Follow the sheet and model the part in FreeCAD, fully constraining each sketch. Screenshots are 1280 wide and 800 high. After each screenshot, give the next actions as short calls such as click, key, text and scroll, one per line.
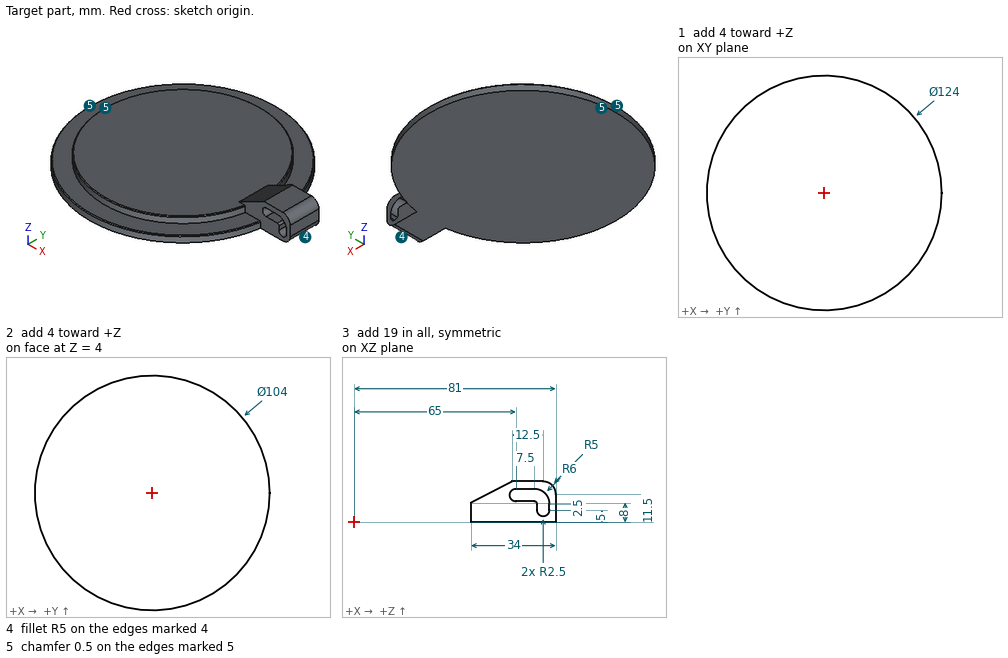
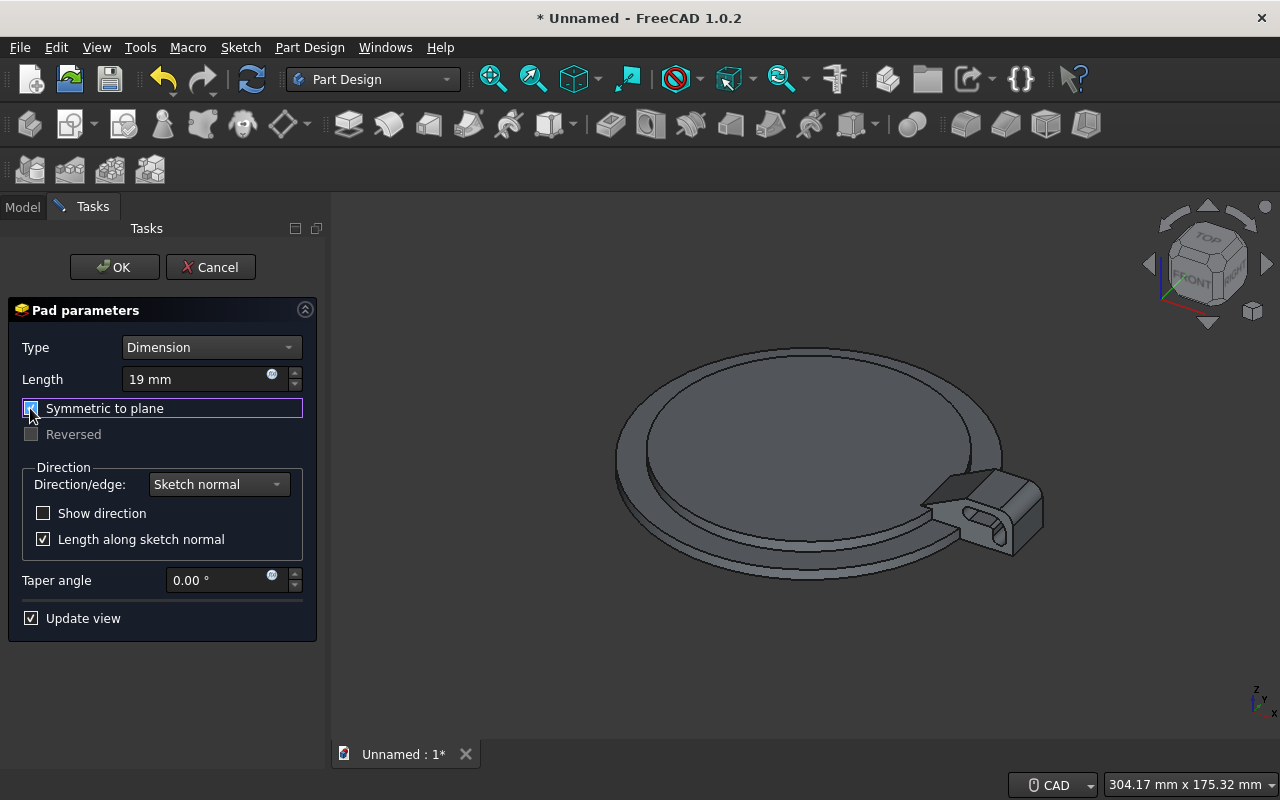
click(115, 267)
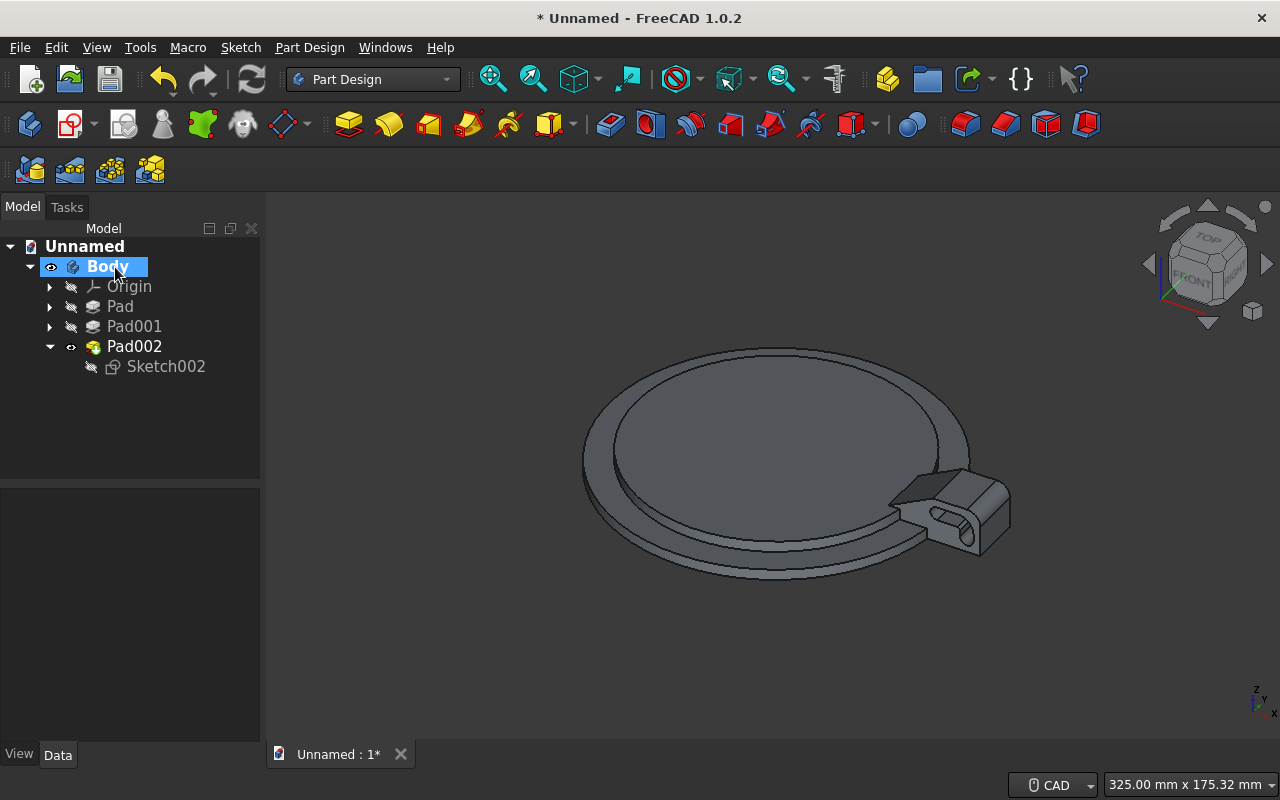
key(0)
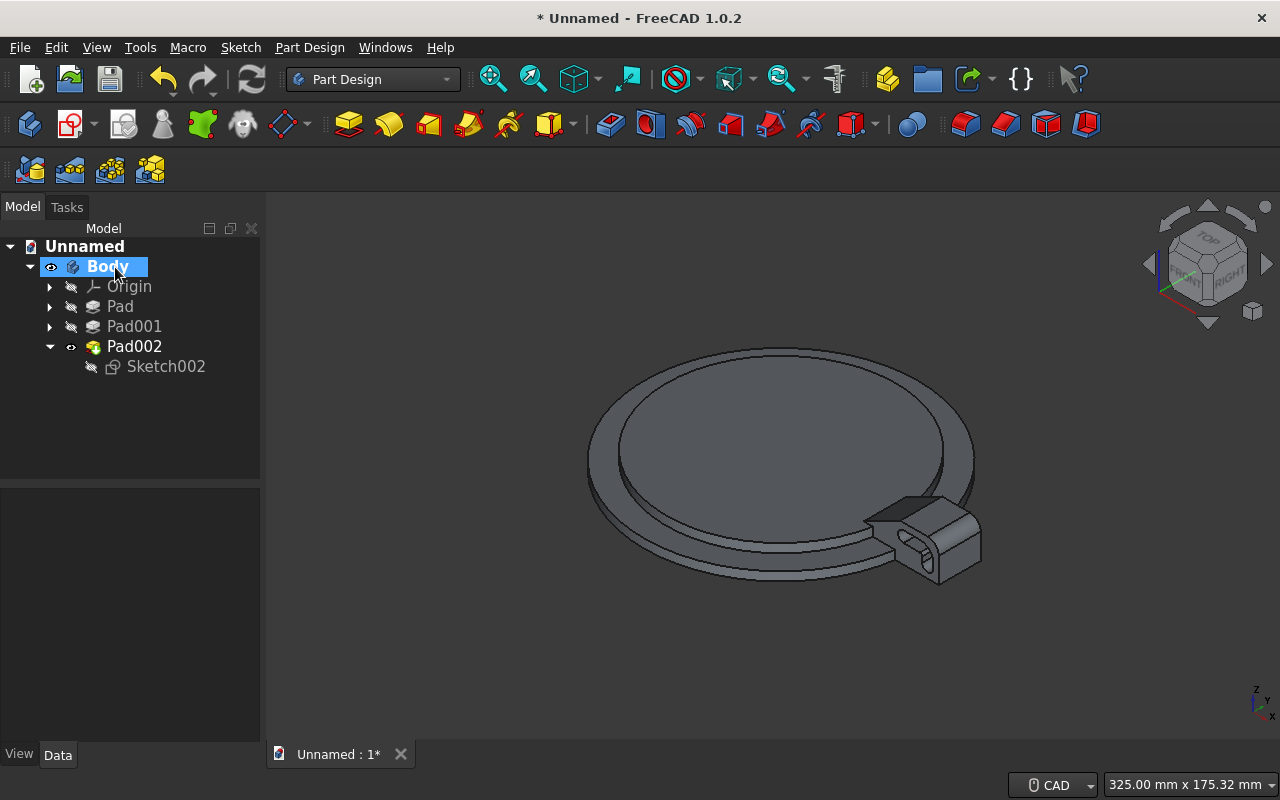
key(2)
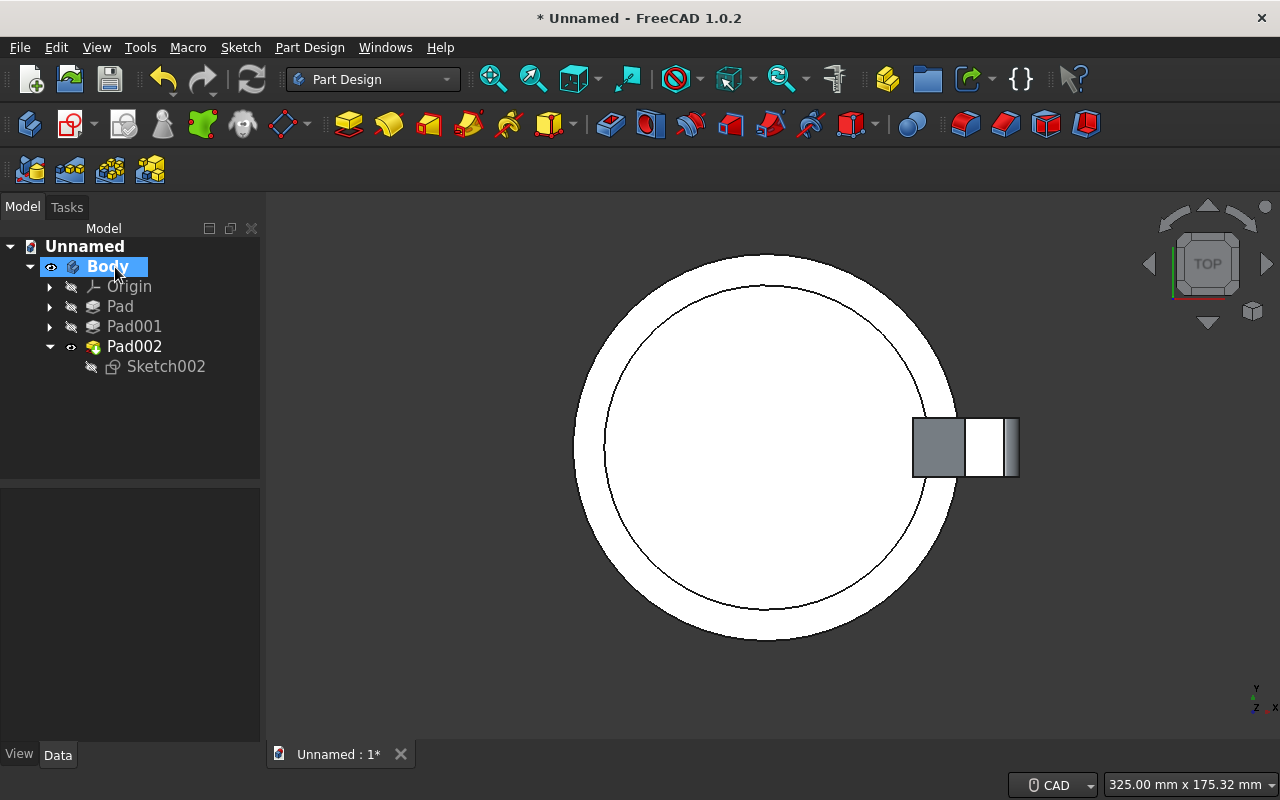
key(1)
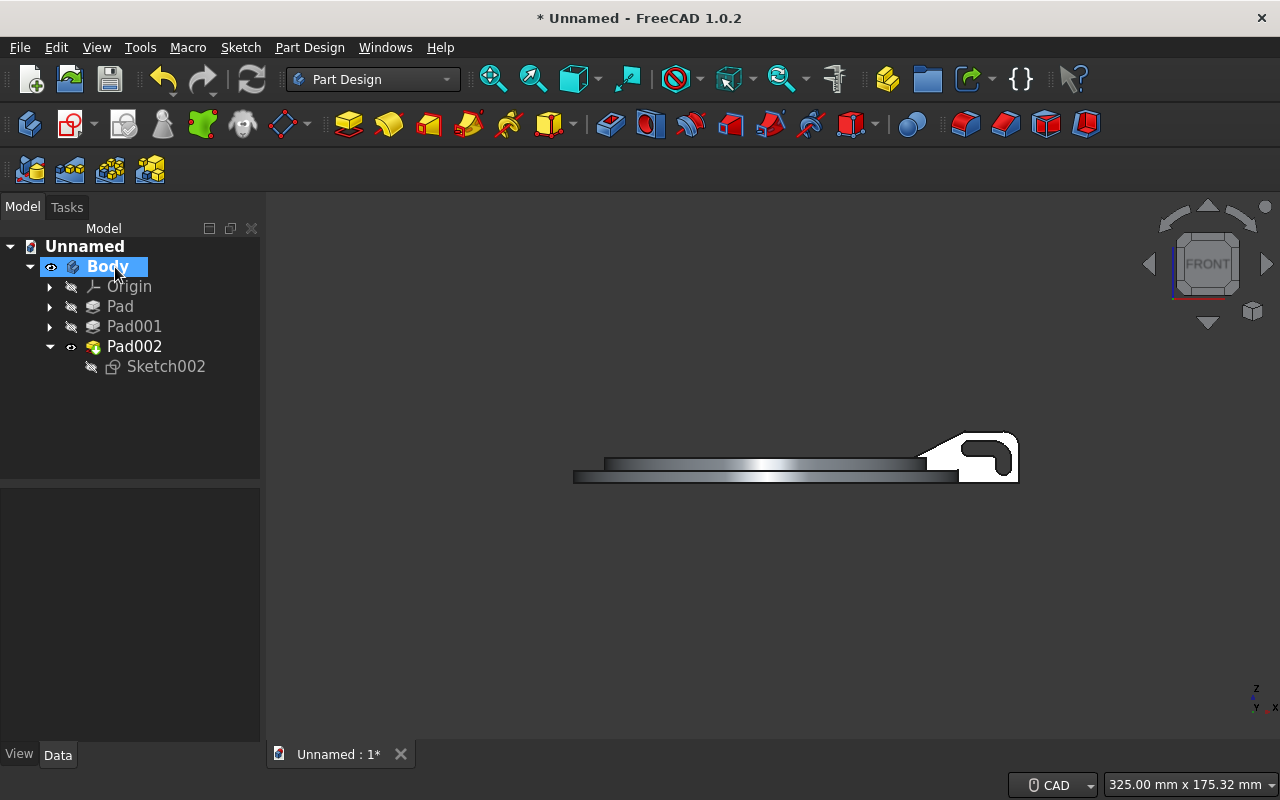
click(494, 80)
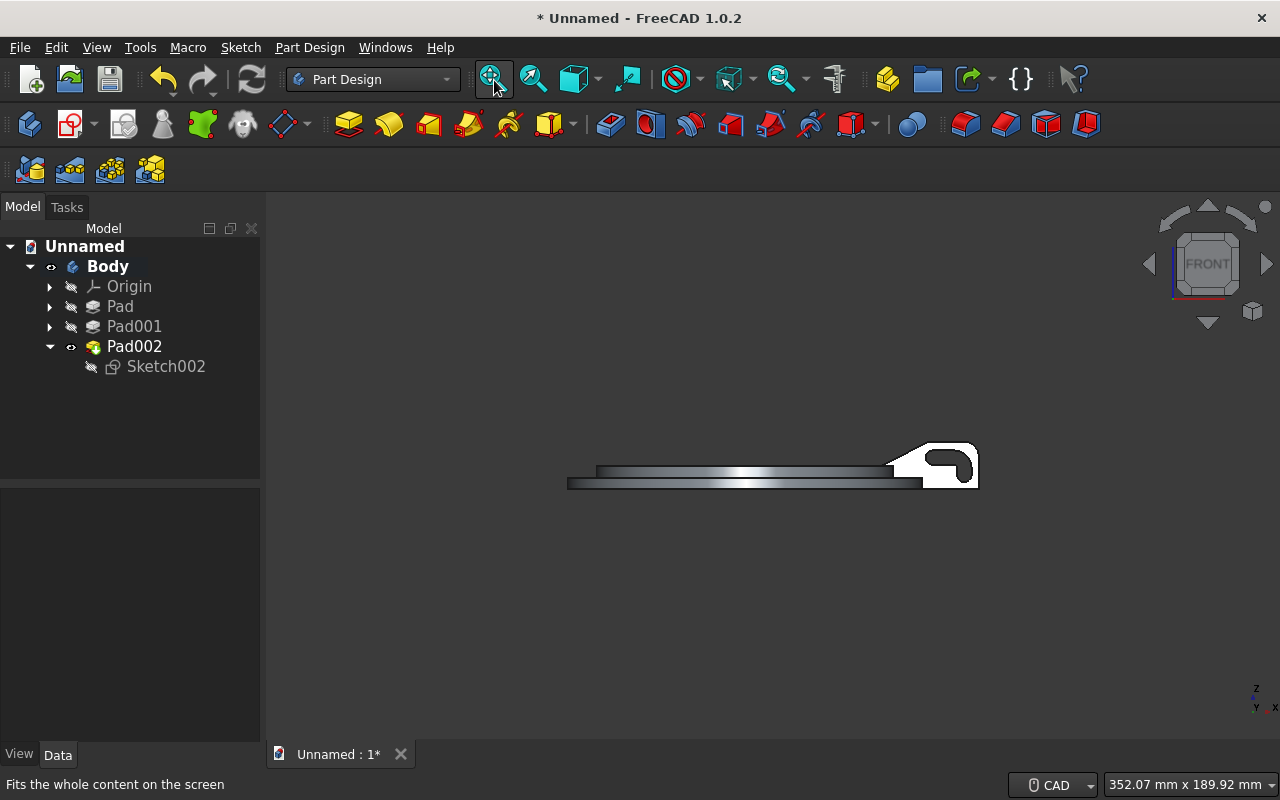
key(3)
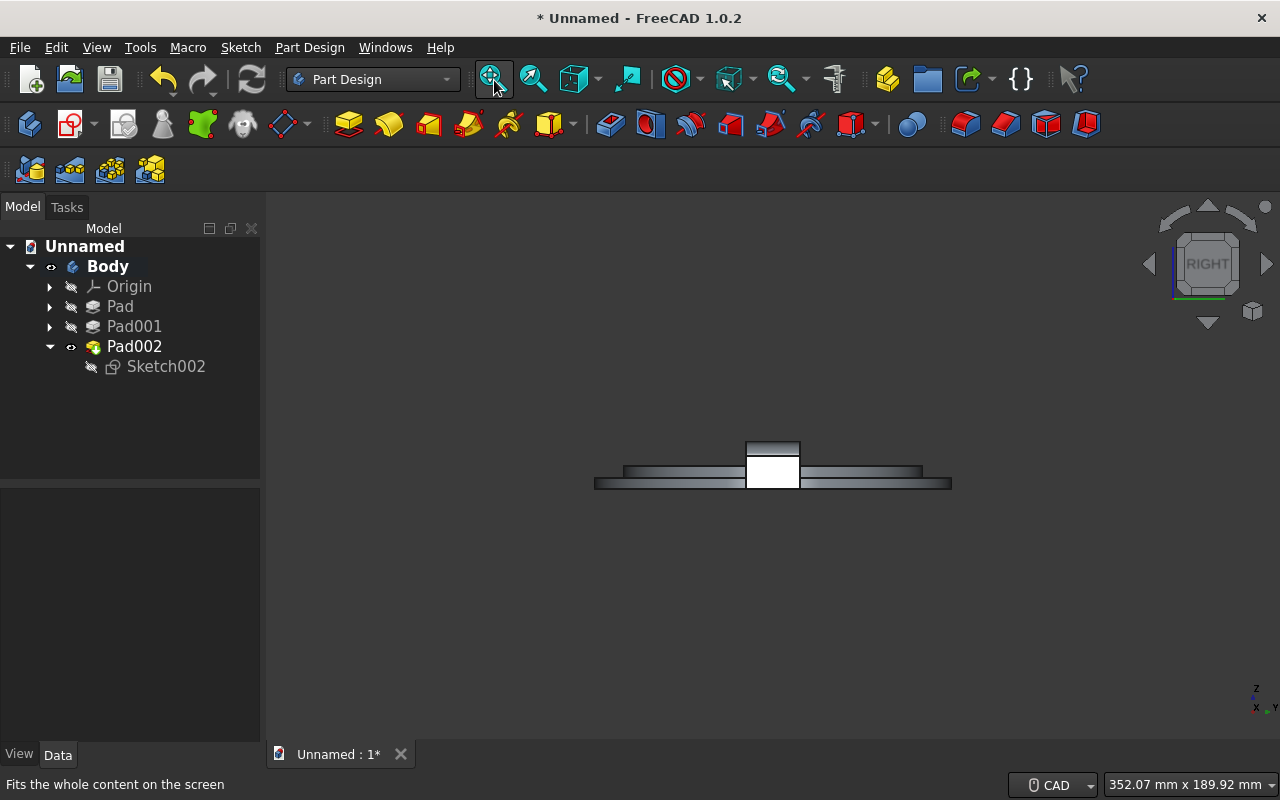
click(494, 80)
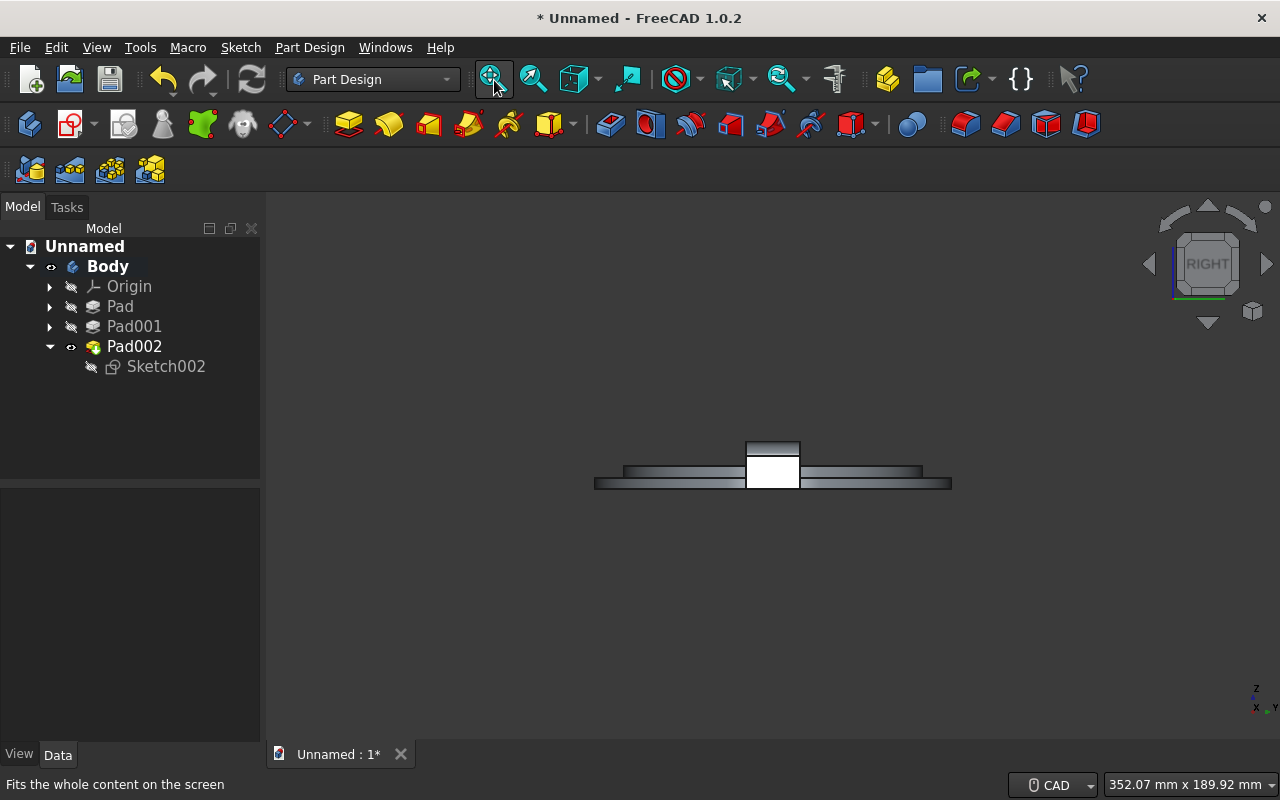
click(773, 488)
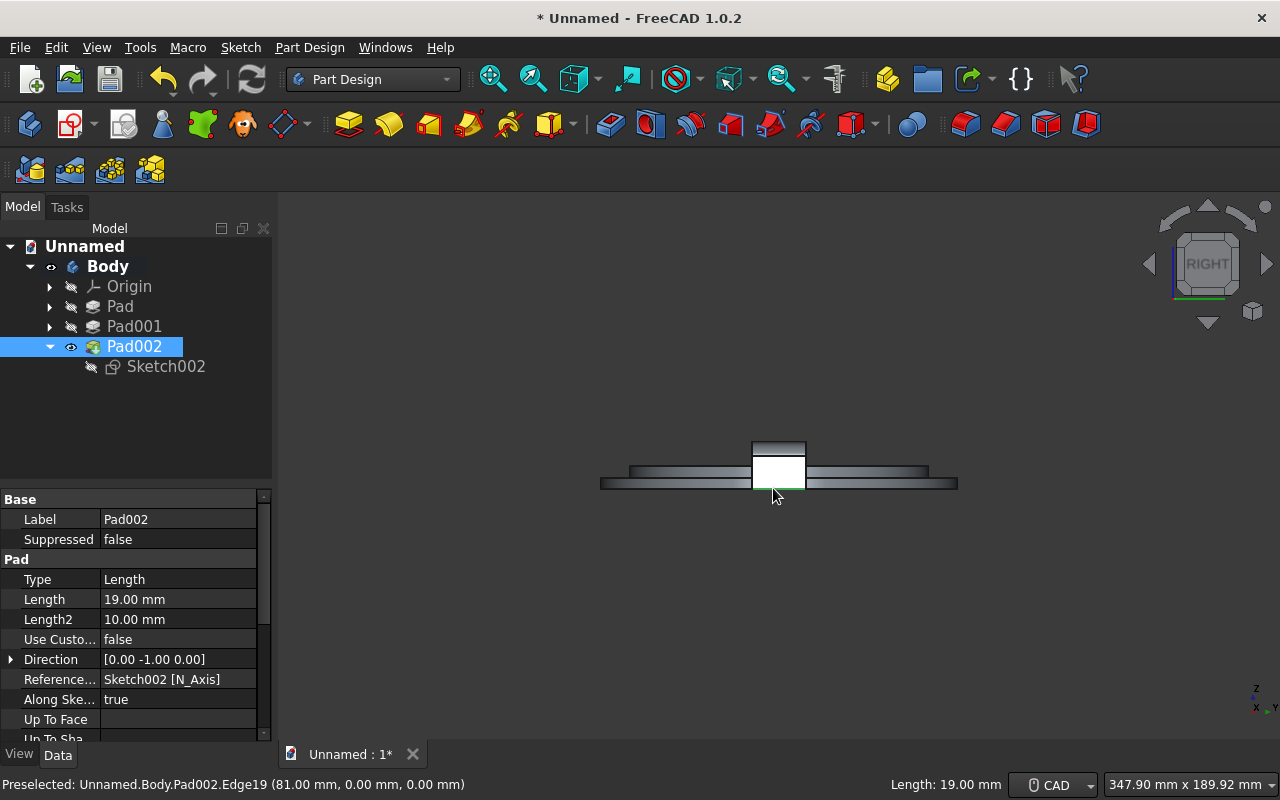
click(966, 124)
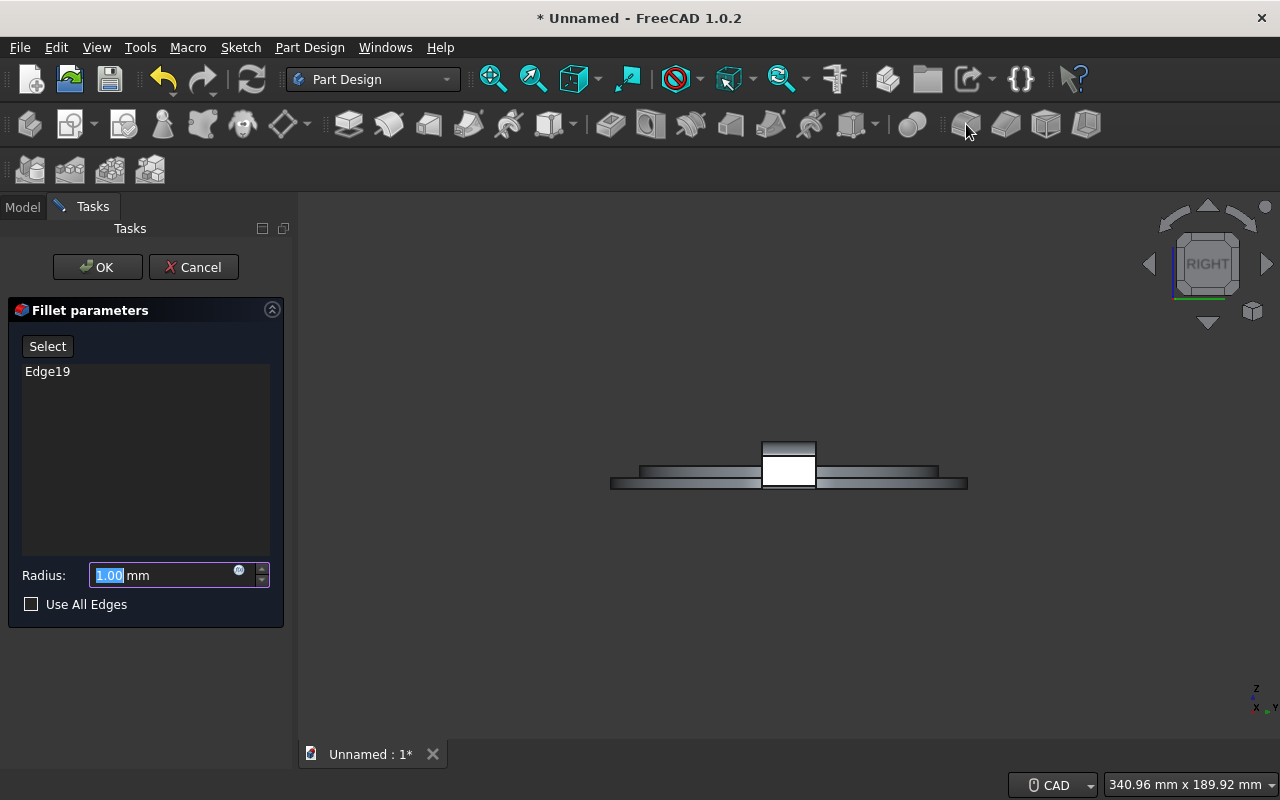
text(5)
key(Tab)